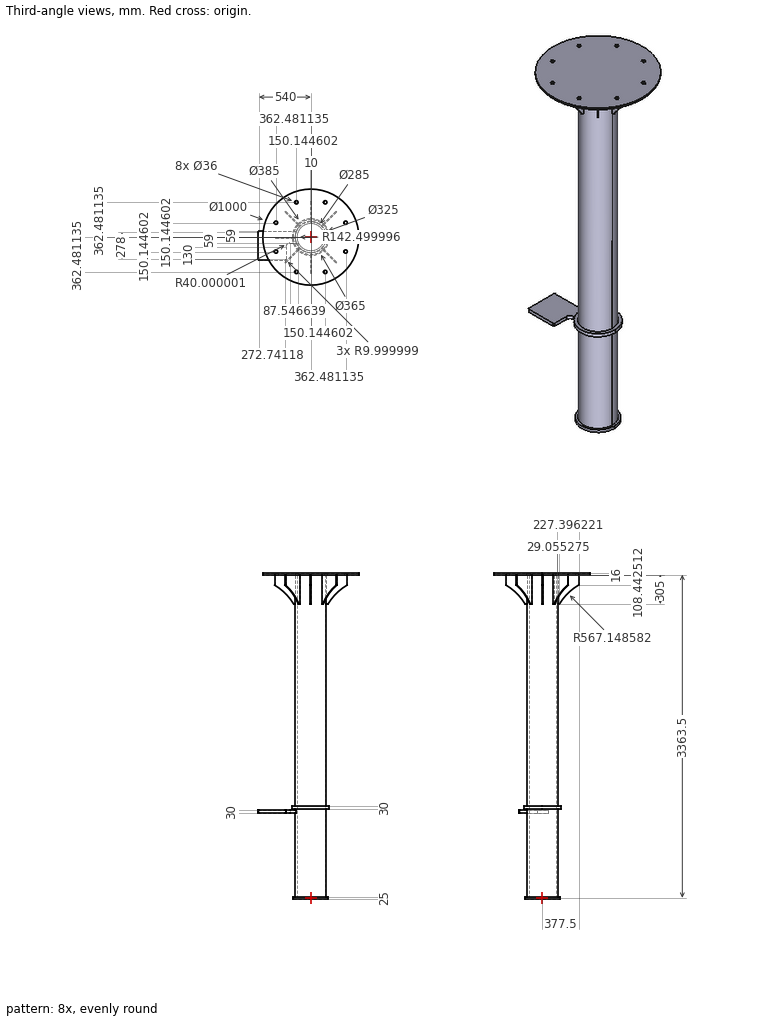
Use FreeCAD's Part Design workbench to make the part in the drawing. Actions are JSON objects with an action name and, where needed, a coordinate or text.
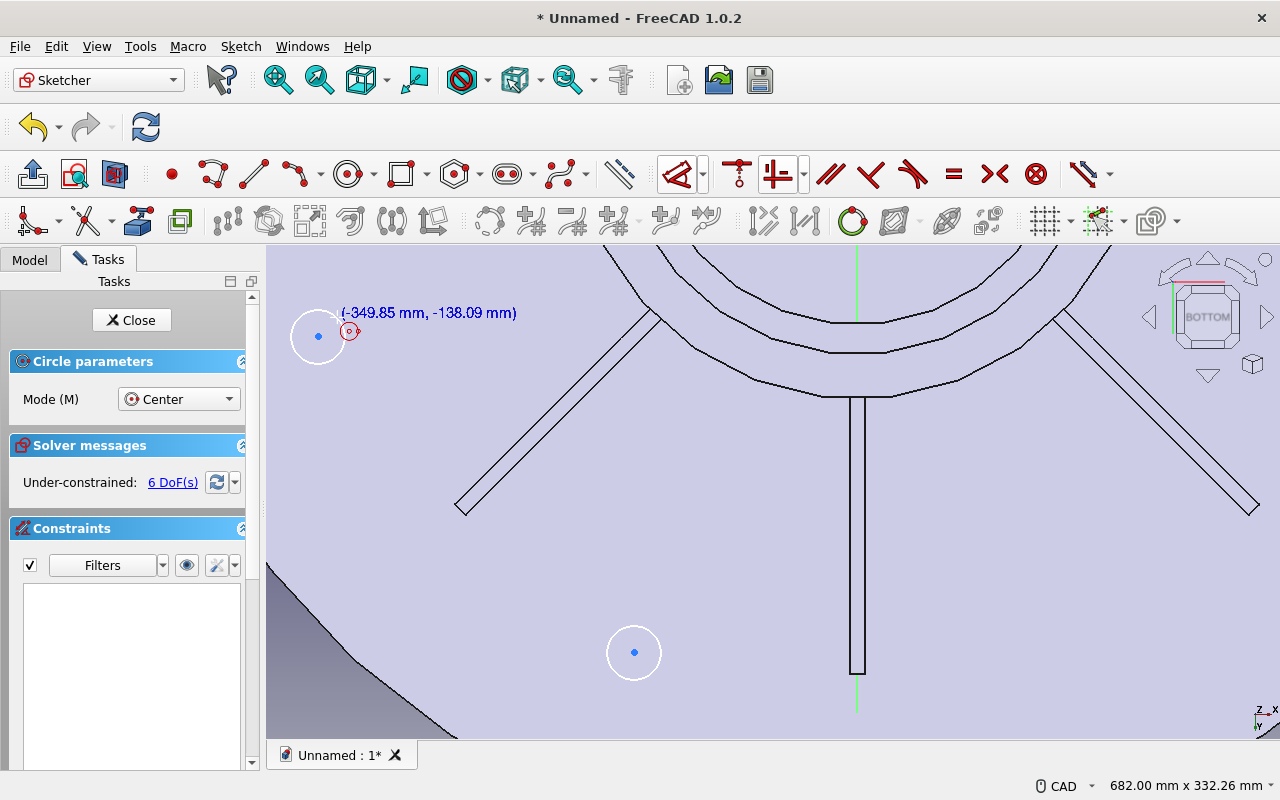
{"action": "scroll", "coordinate": [639, 655], "scroll_direction": "down", "scroll_amount": 6}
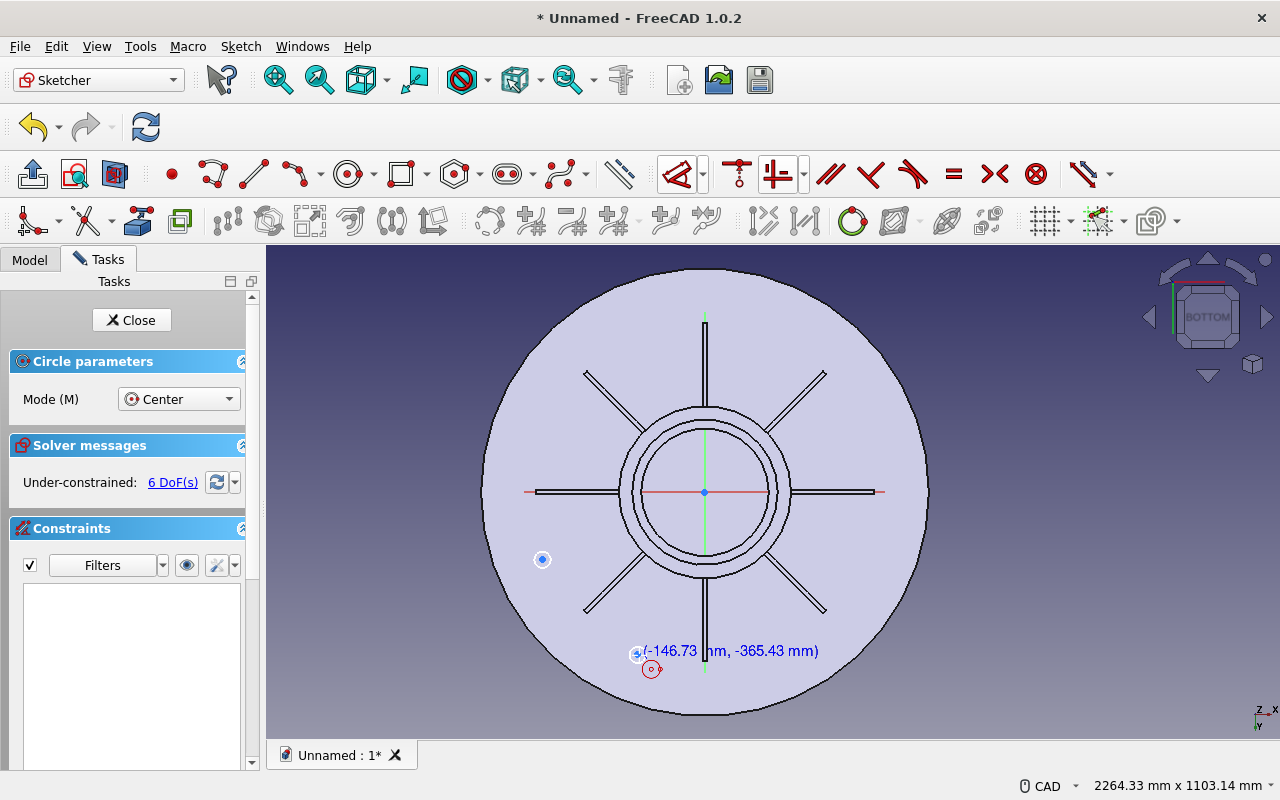
{"action": "scroll", "coordinate": [543, 425], "scroll_direction": "up", "scroll_amount": 6}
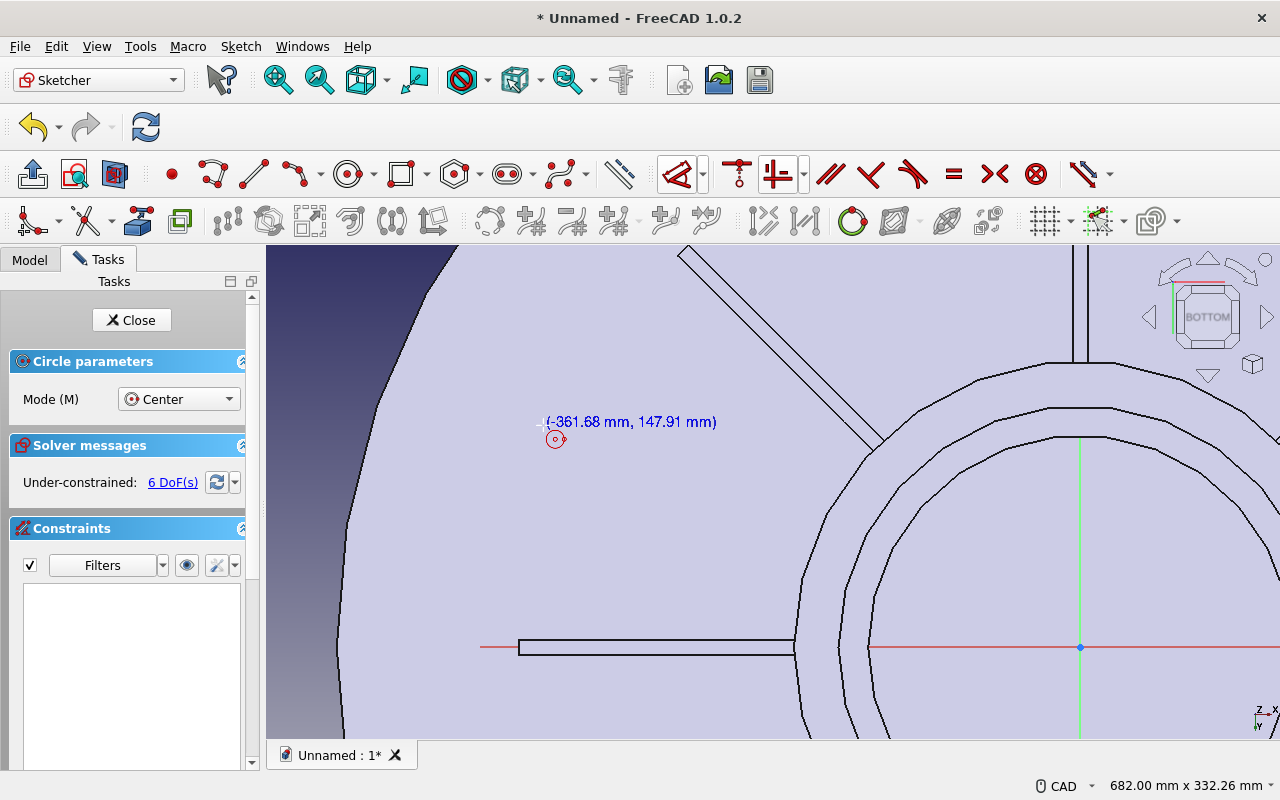
{"action": "left_click", "coordinate": [541, 424]}
{"action": "left_click", "coordinate": [560, 405]}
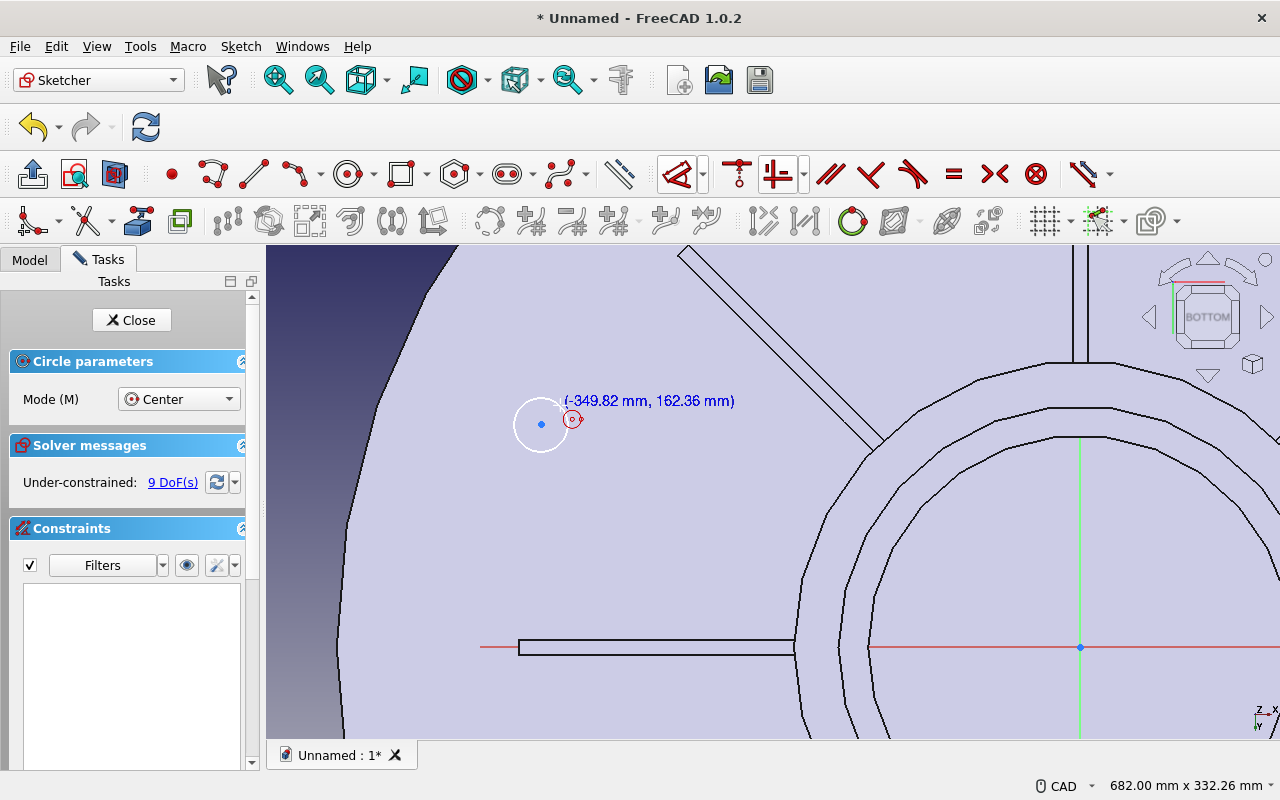
{"action": "scroll", "coordinate": [543, 425], "scroll_direction": "down", "scroll_amount": 6}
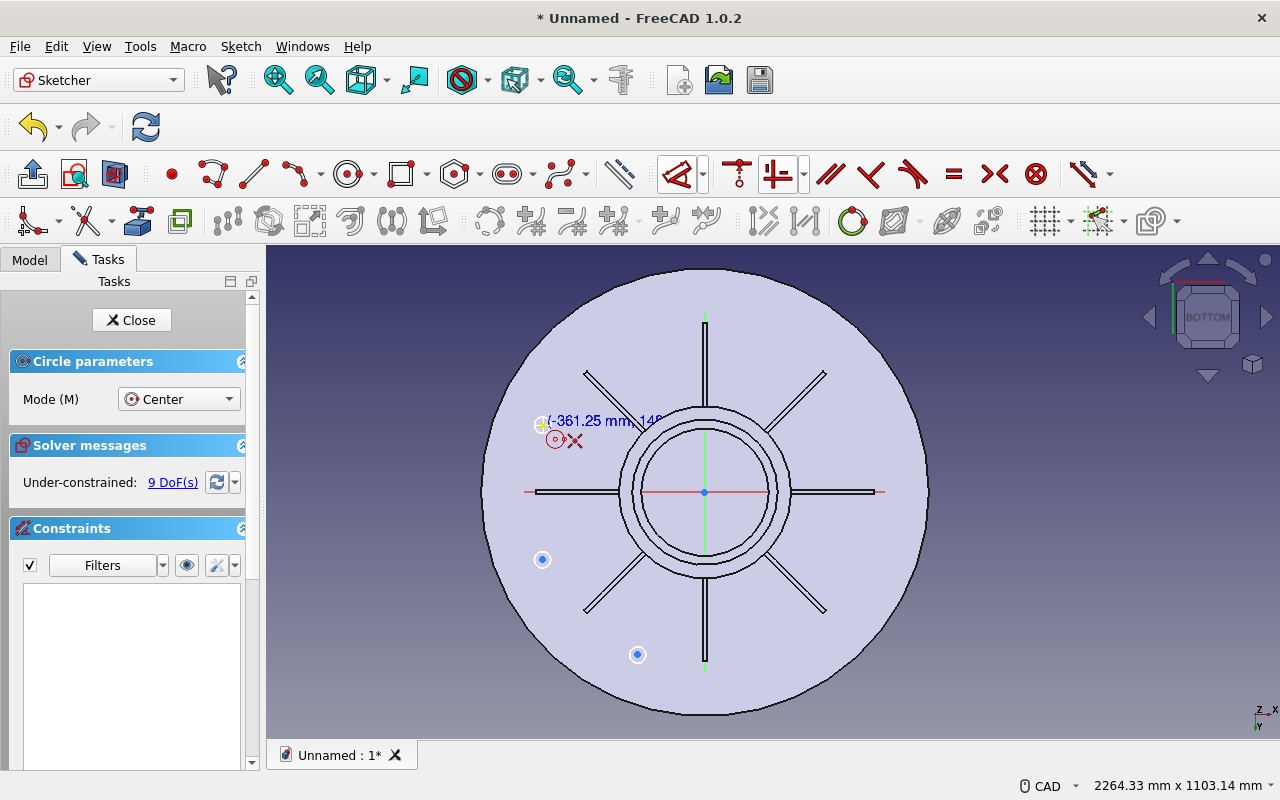
{"action": "scroll", "coordinate": [638, 330], "scroll_direction": "up", "scroll_amount": 6}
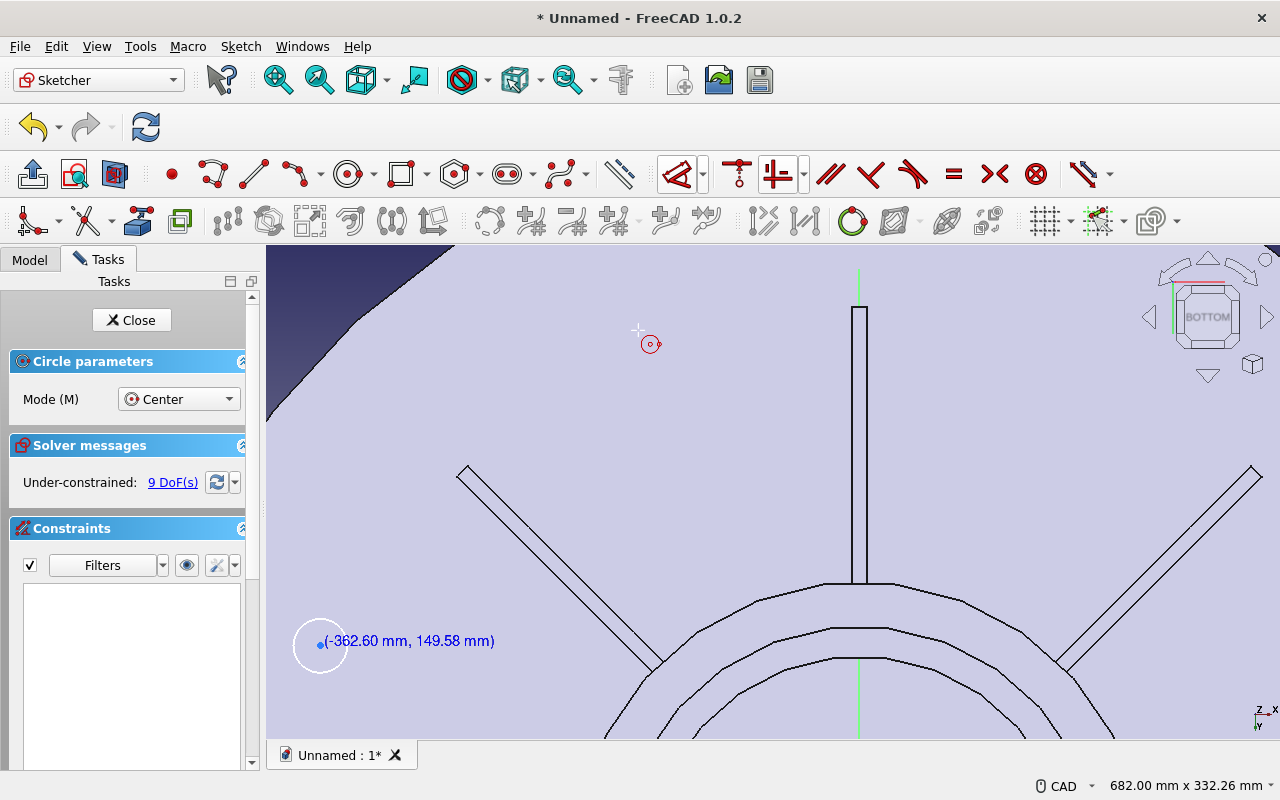
{"action": "left_click", "coordinate": [636, 329]}
{"action": "left_click", "coordinate": [655, 310]}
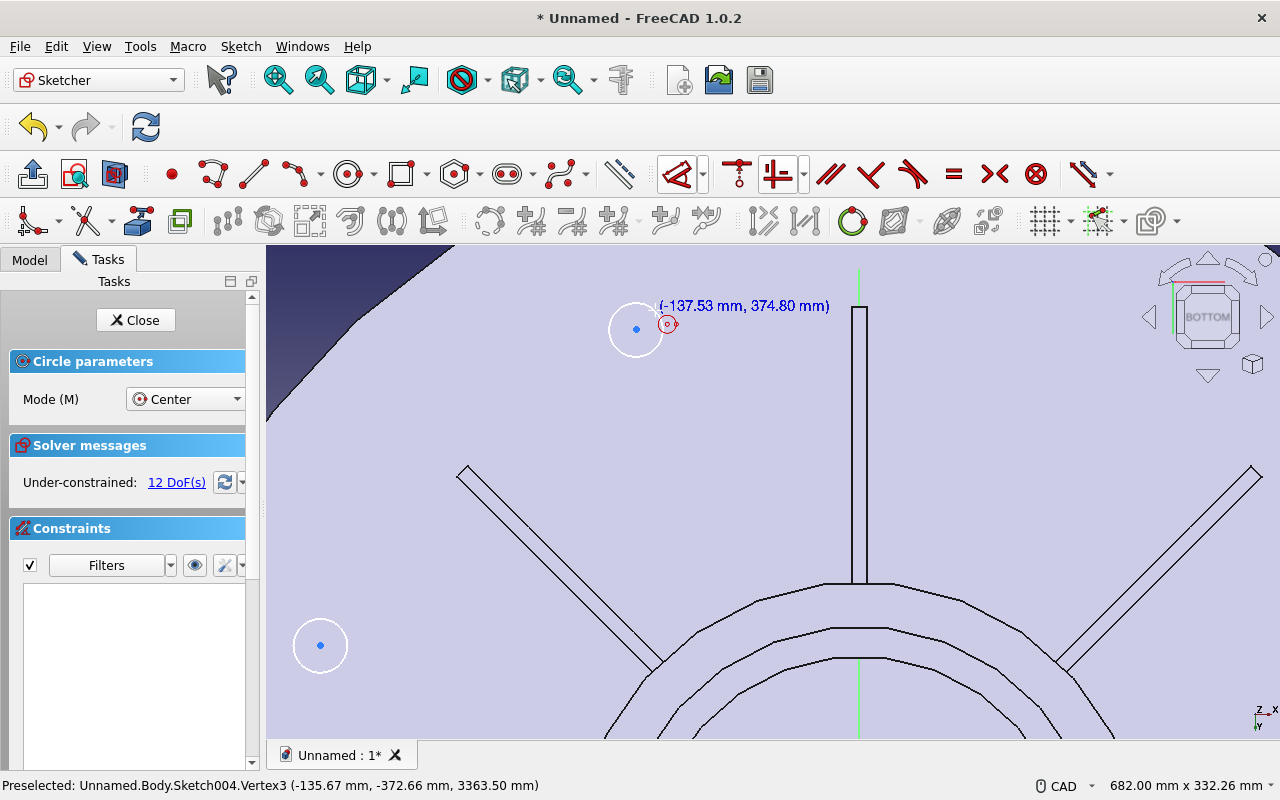
{"action": "left_click", "coordinate": [1083, 329]}
{"action": "left_click", "coordinate": [1102, 310]}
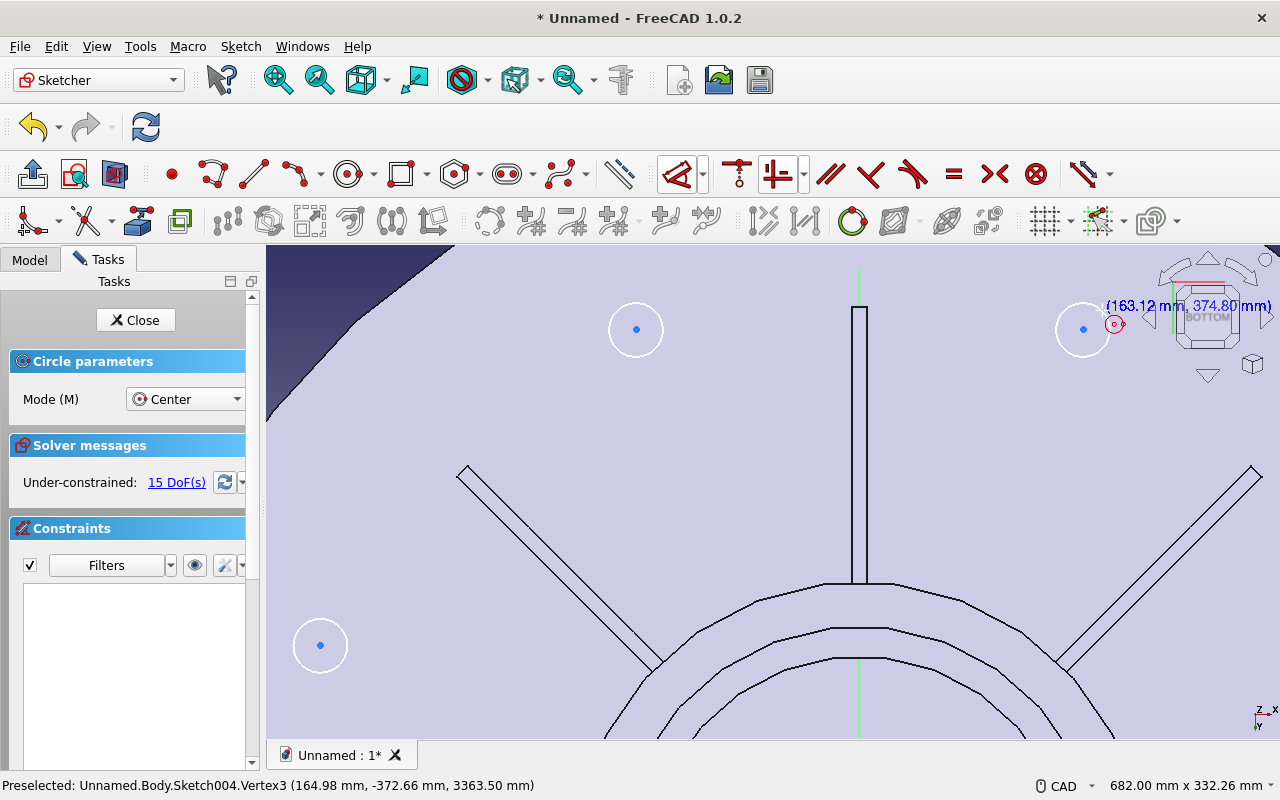
{"action": "scroll", "coordinate": [638, 330], "scroll_direction": "down", "scroll_amount": 6}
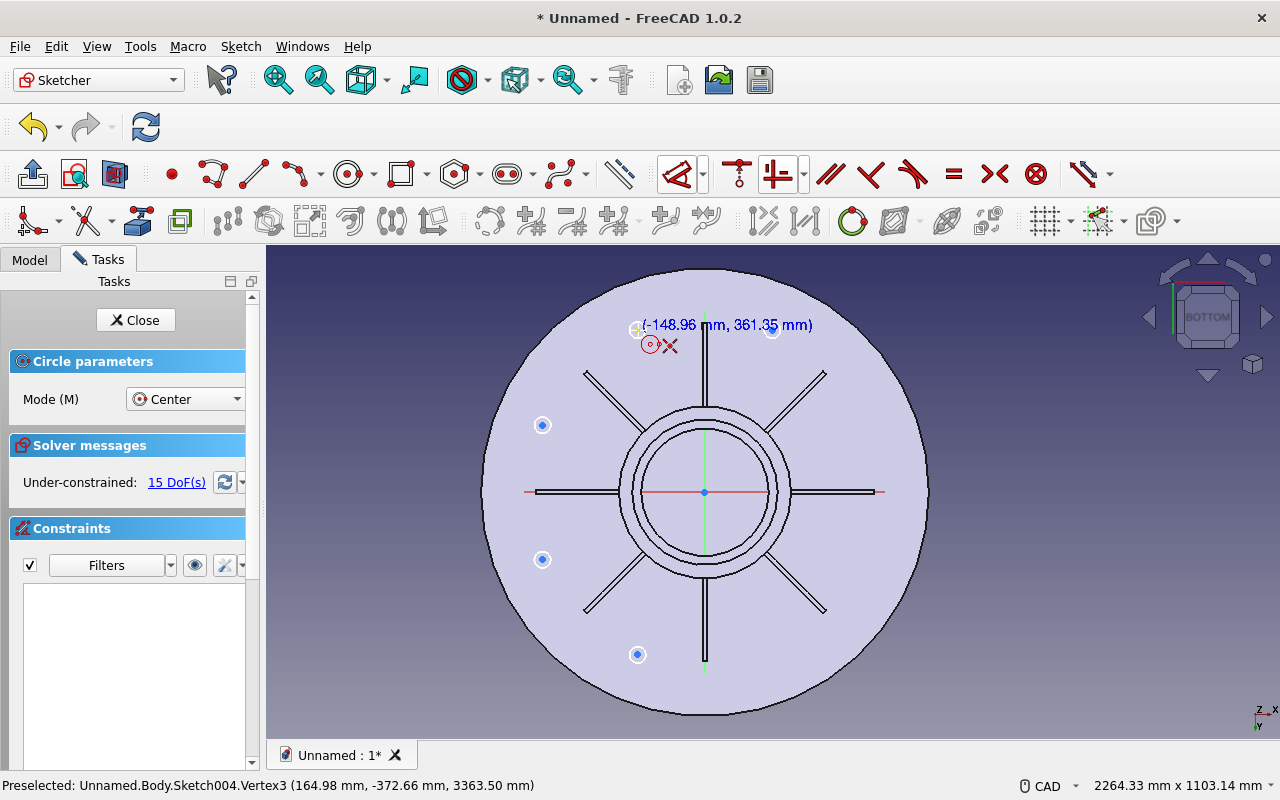
{"action": "scroll", "coordinate": [867, 425], "scroll_direction": "up", "scroll_amount": 6}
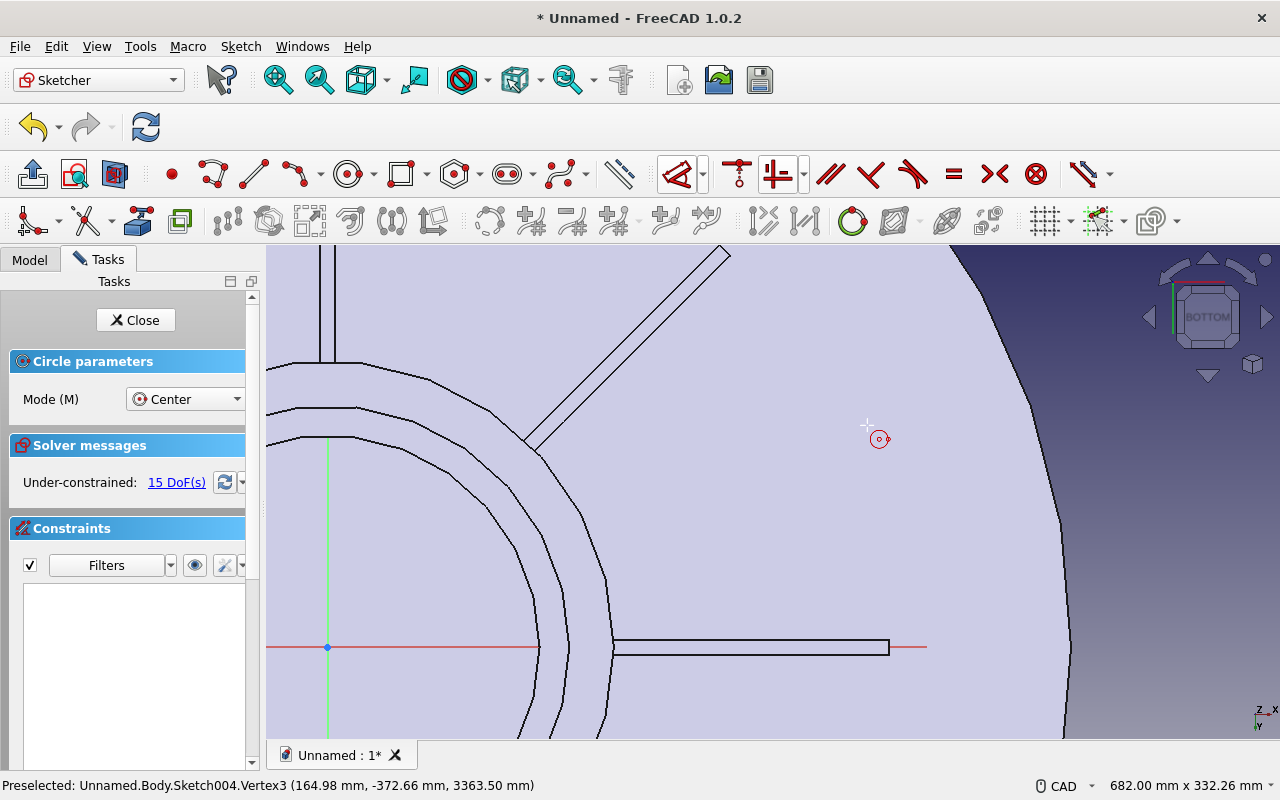
{"action": "left_click", "coordinate": [867, 424]}
{"action": "left_click", "coordinate": [886, 405]}